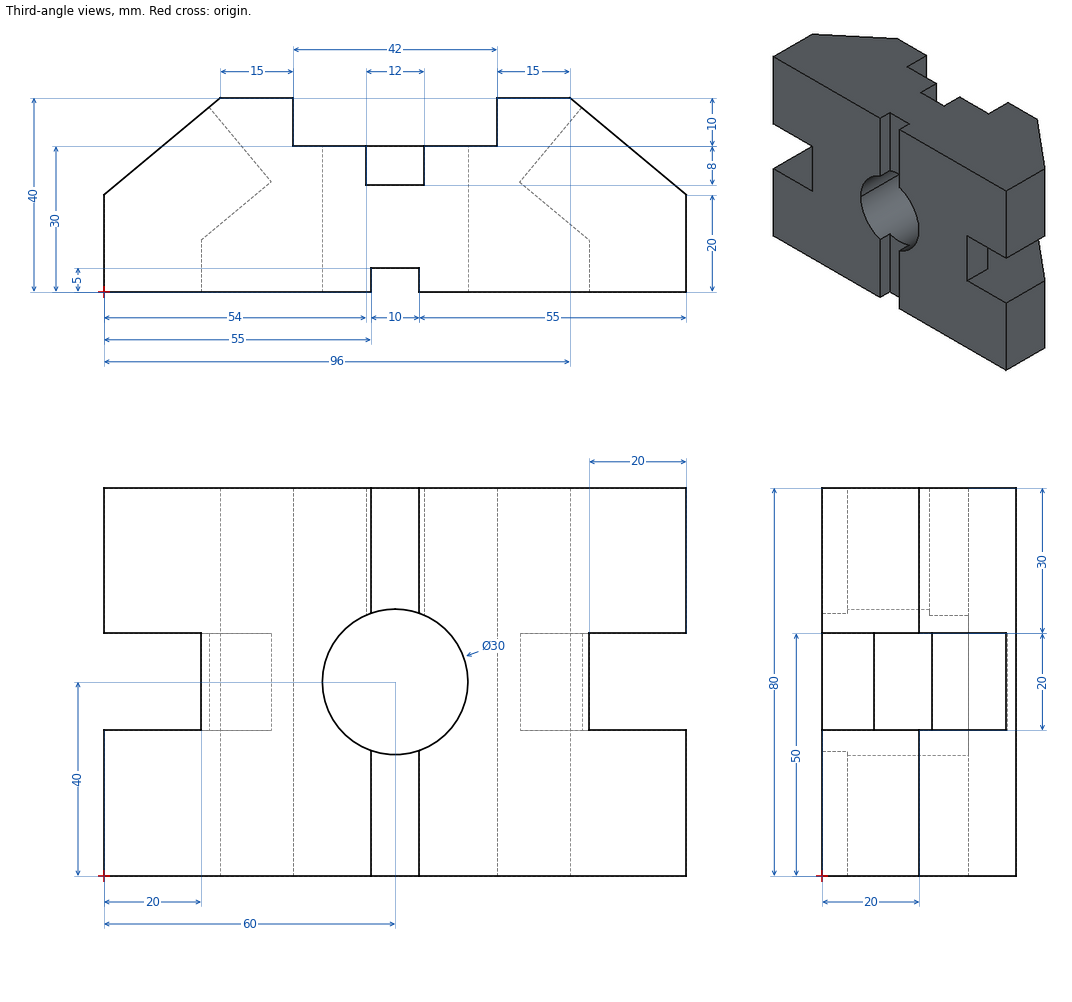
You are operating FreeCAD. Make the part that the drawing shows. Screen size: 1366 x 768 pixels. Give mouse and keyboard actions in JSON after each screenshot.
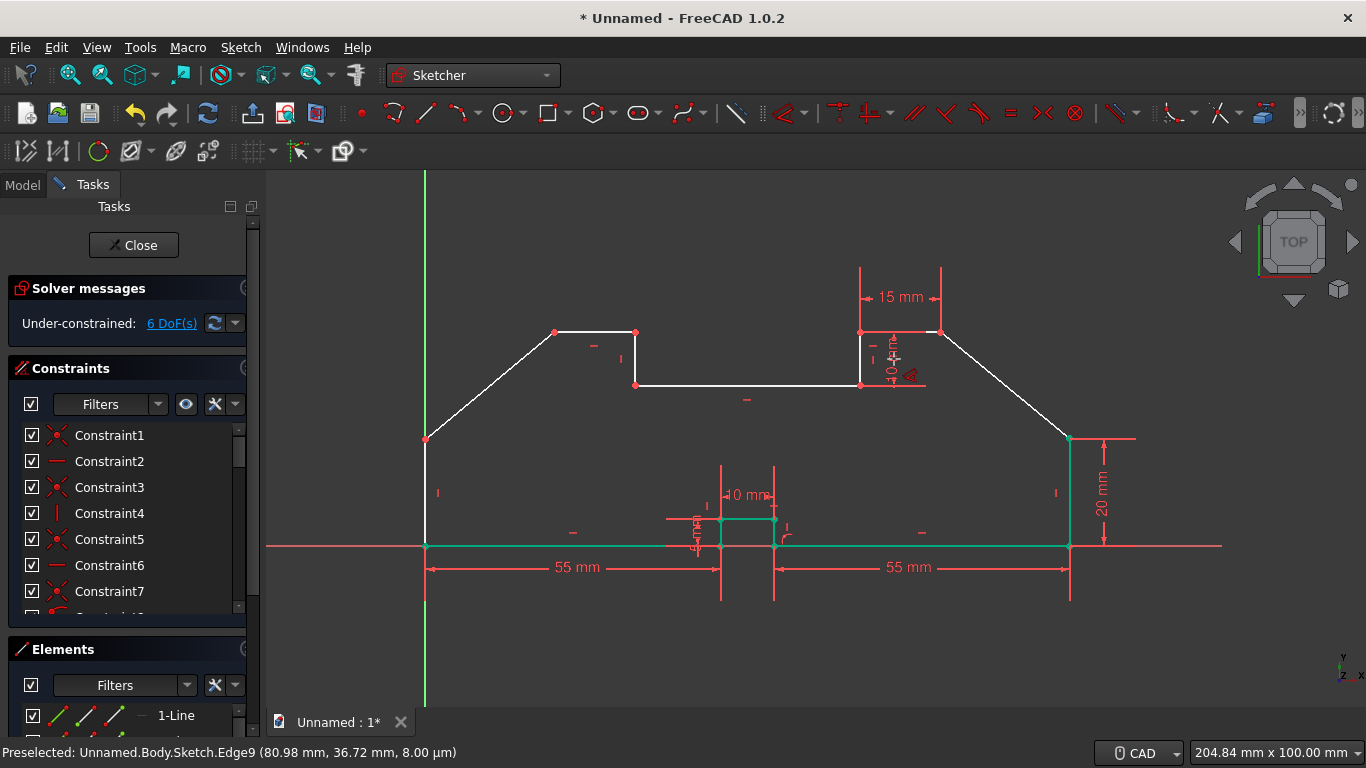
{"action": "left_click", "coordinate": [793, 386]}
{"action": "left_click", "coordinate": [748, 352]}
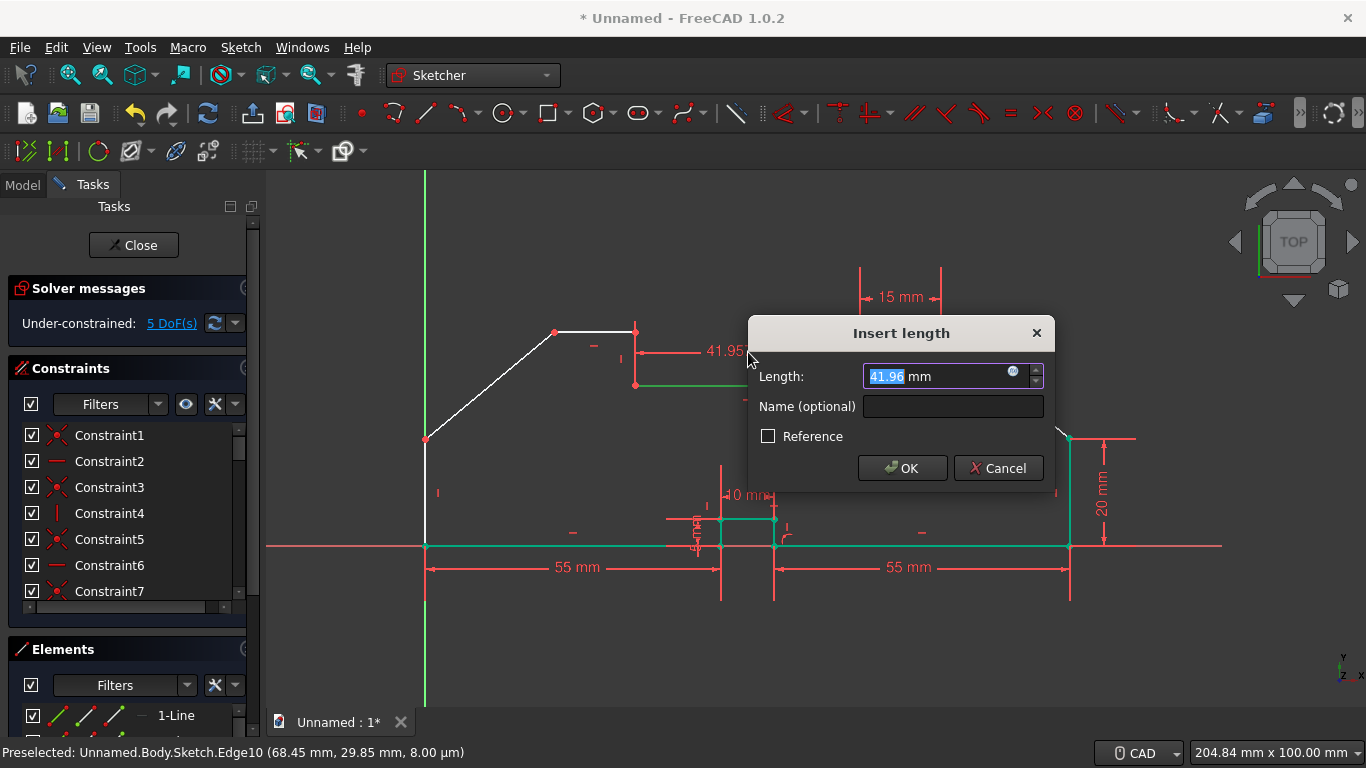
{"action": "type", "text": "42"}
{"action": "key", "text": "Return"}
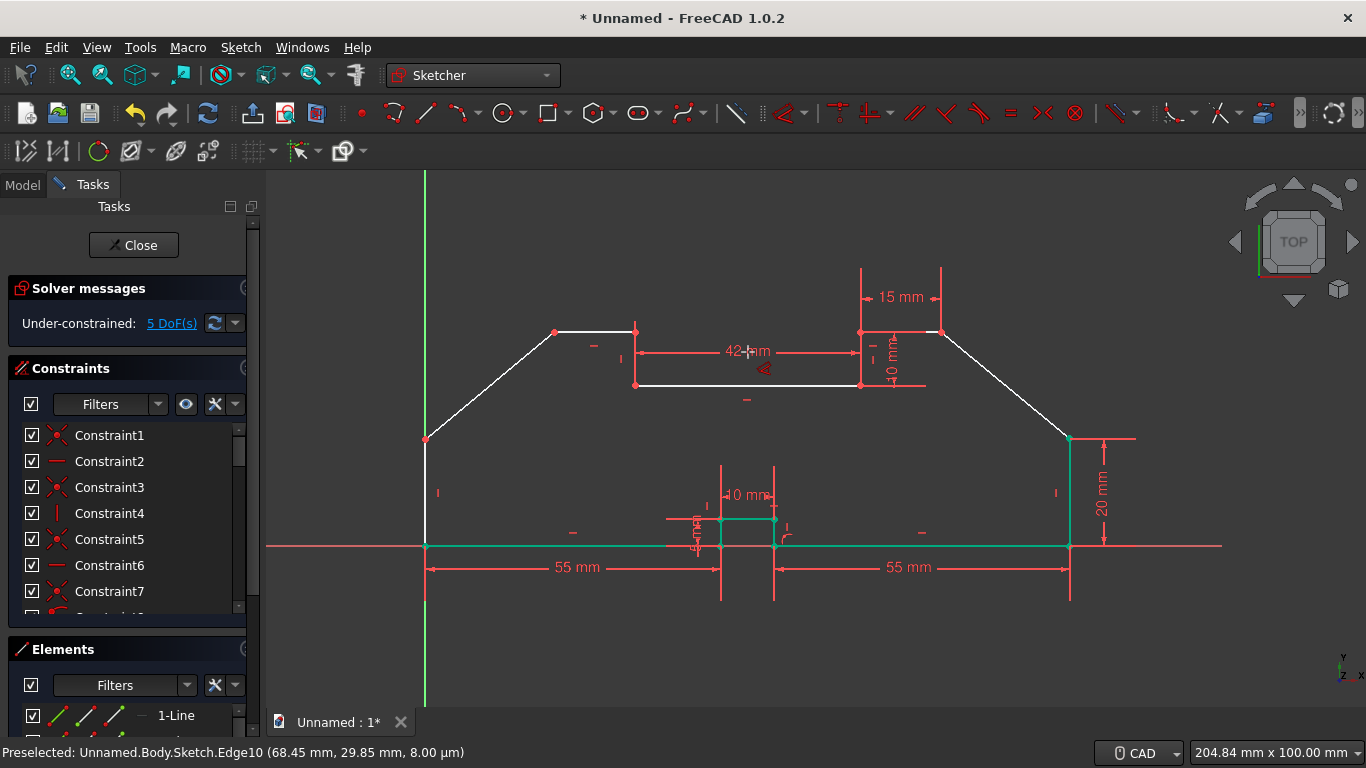
{"action": "left_click", "coordinate": [635, 370]}
{"action": "left_click", "coordinate": [601, 359]}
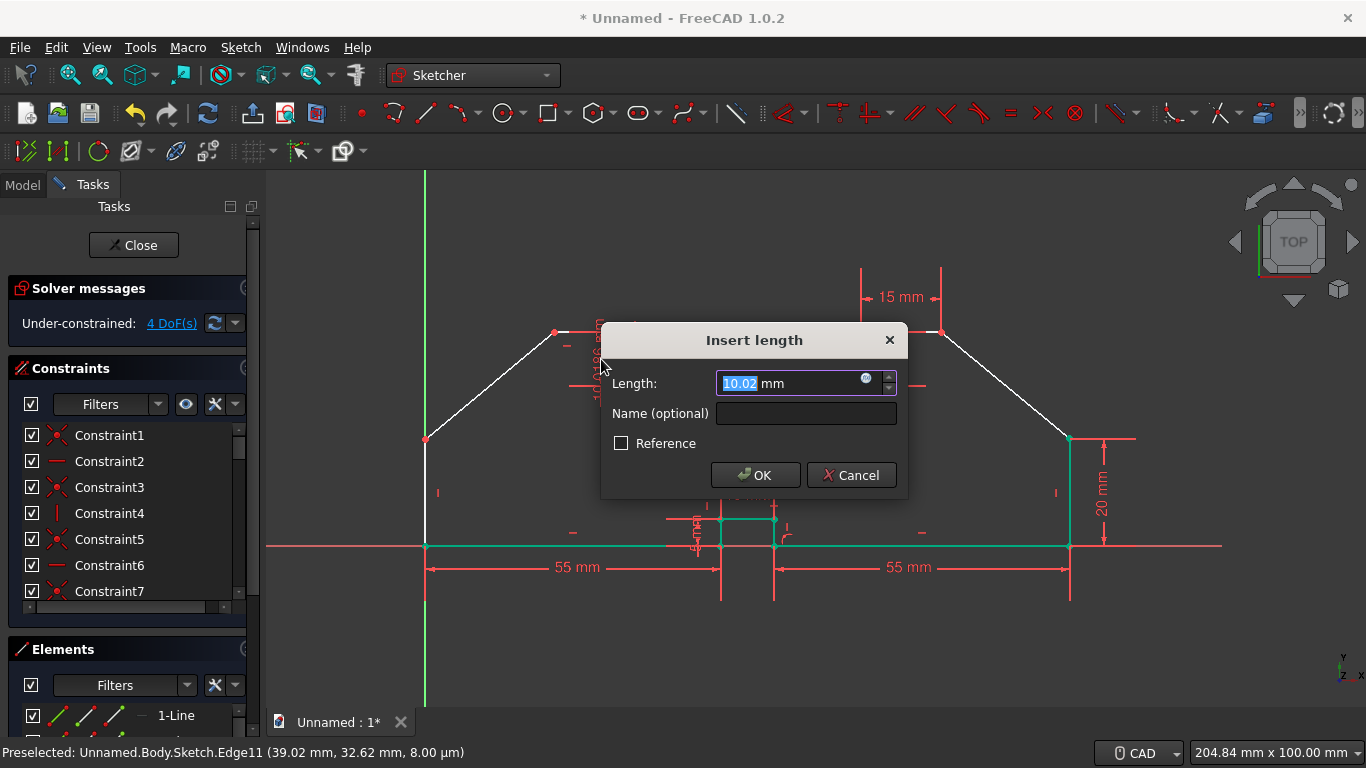
{"action": "type", "text": "10"}
{"action": "key", "text": "Return"}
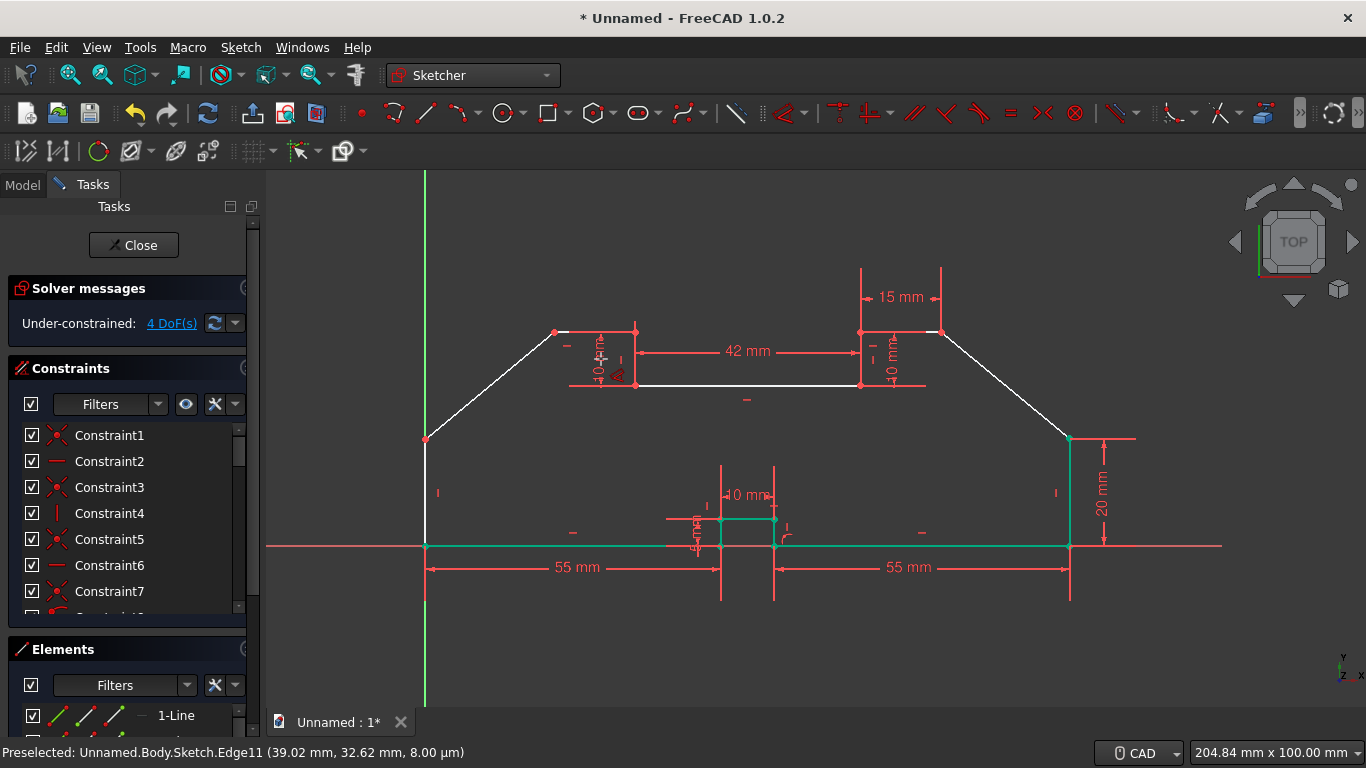
{"action": "left_click", "coordinate": [611, 332]}
{"action": "left_click", "coordinate": [595, 298]}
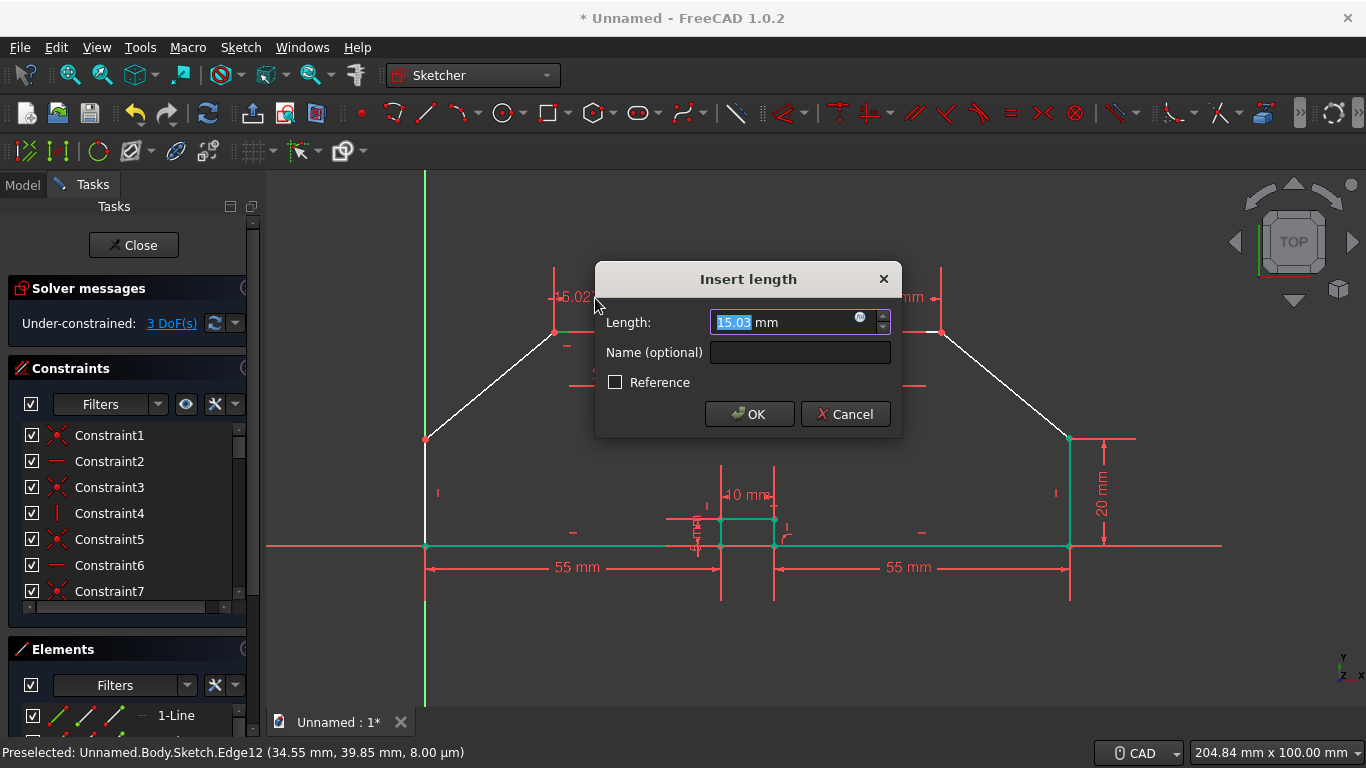
{"action": "type", "text": "15"}
{"action": "key", "text": "Return"}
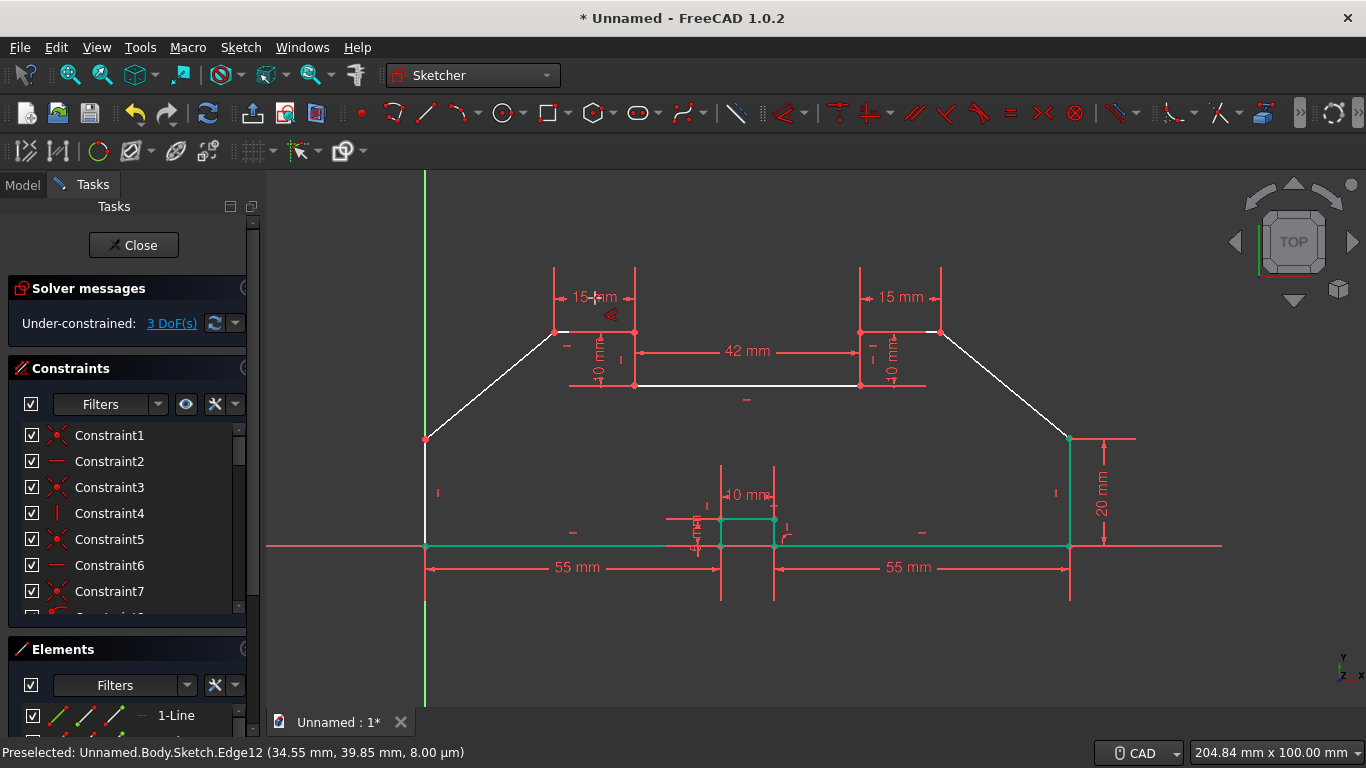
{"action": "left_click", "coordinate": [425, 472]}
{"action": "left_click", "coordinate": [391, 493]}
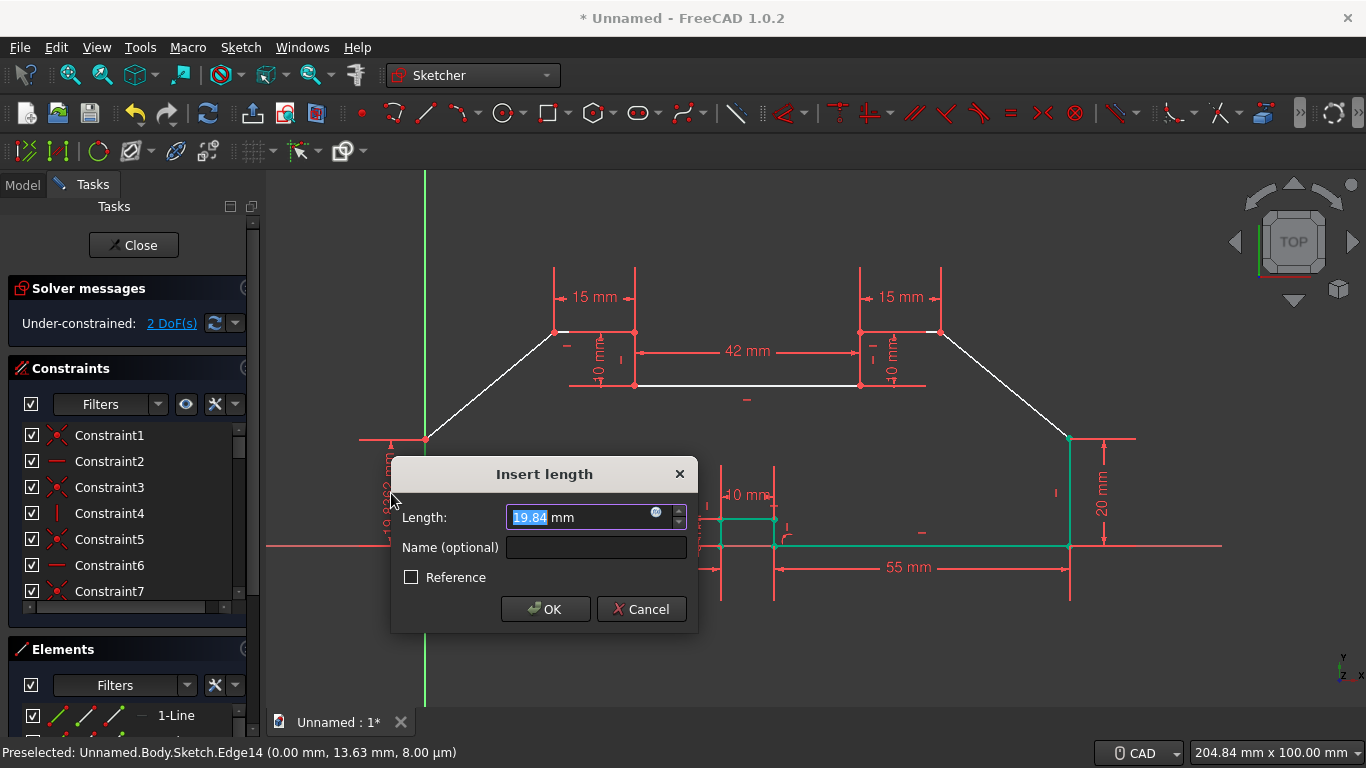
{"action": "type", "text": "20"}
{"action": "key", "text": "Return"}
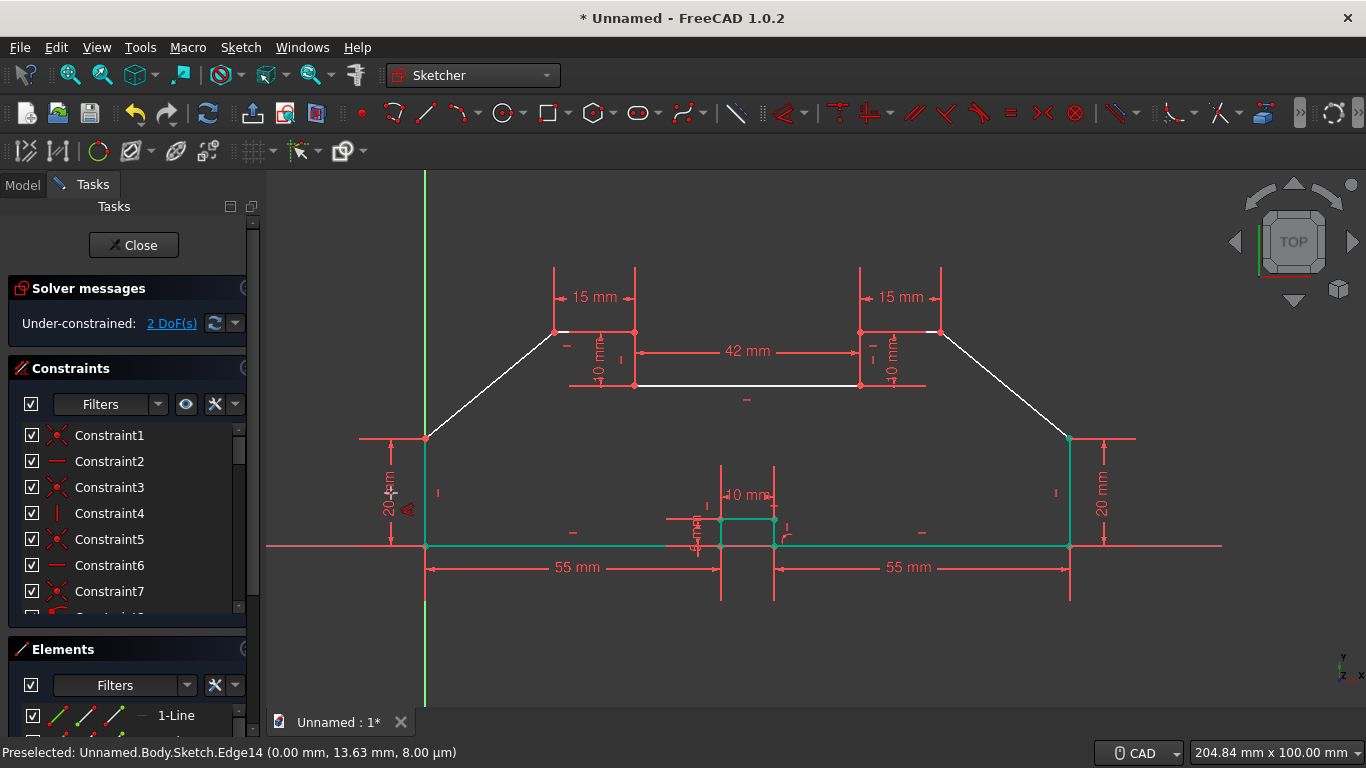
{"action": "left_click", "coordinate": [941, 332]}
{"action": "left_click", "coordinate": [683, 580]}